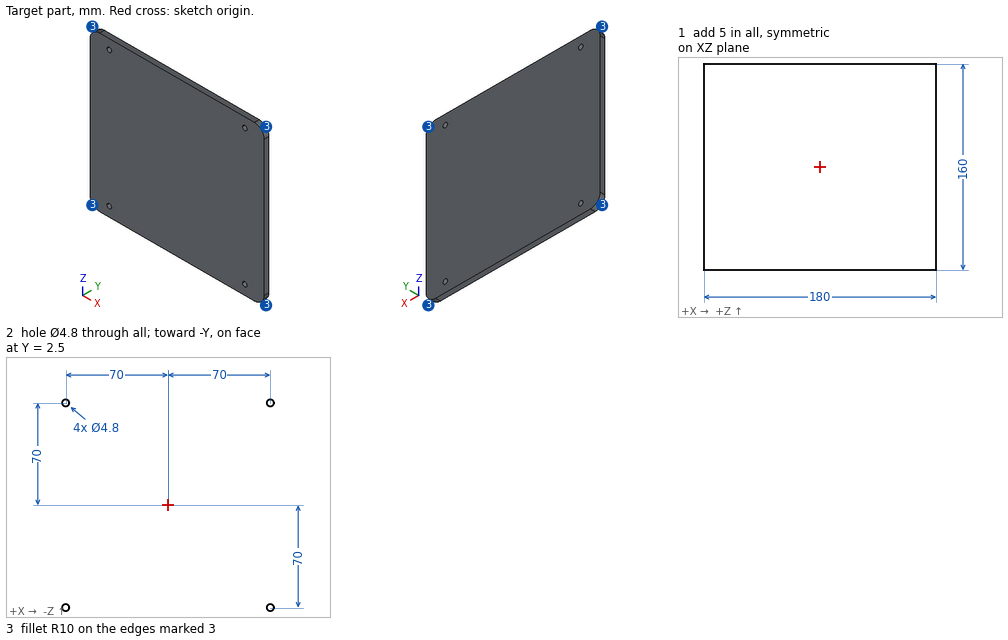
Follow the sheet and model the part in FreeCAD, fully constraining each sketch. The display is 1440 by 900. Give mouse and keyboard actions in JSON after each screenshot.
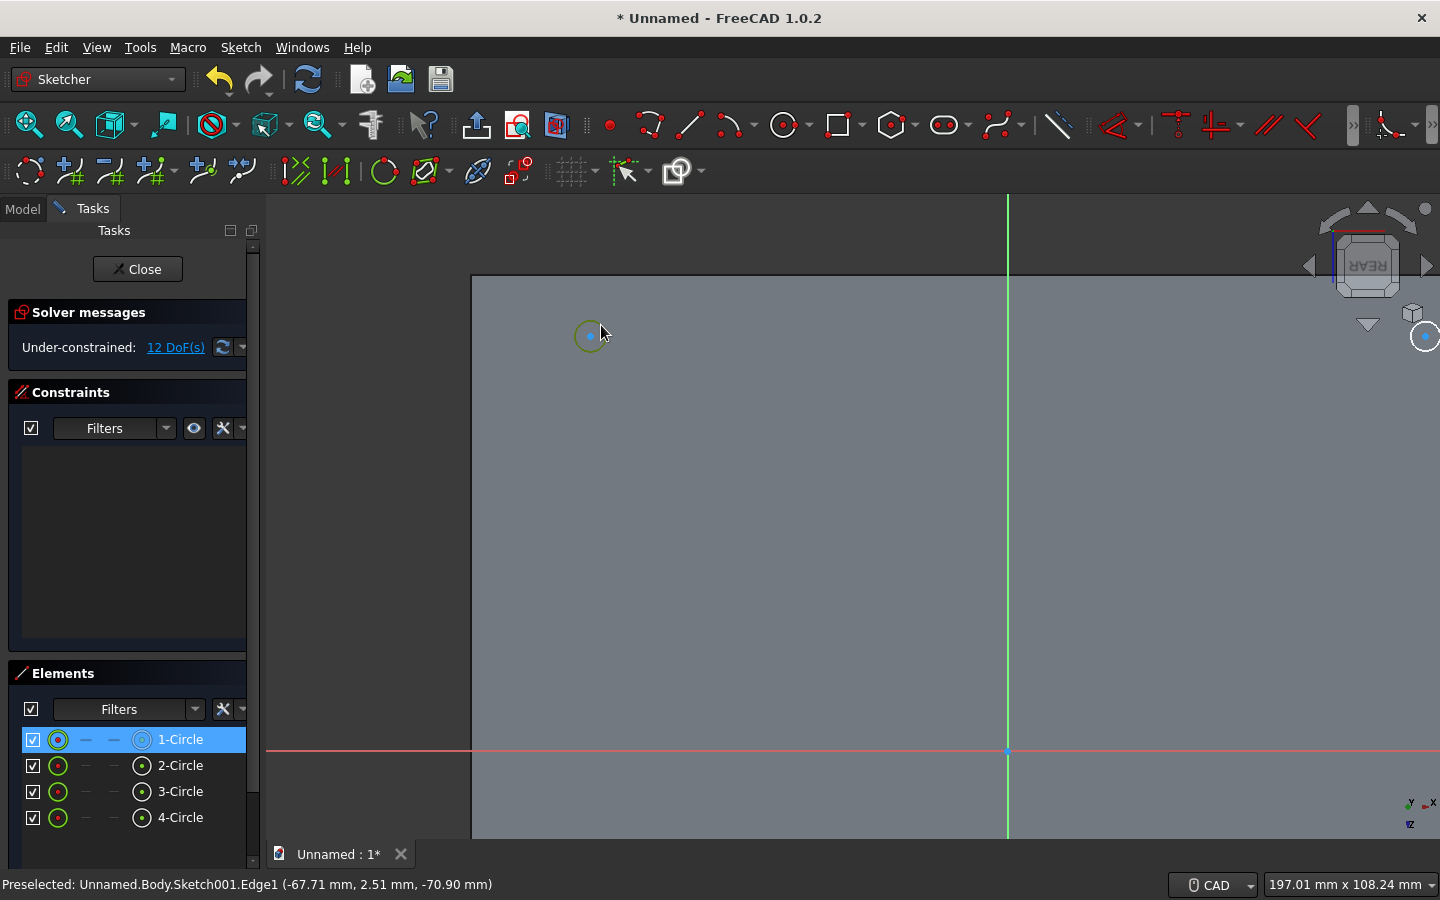
{"action": "scroll", "coordinate": [603, 325], "scroll_direction": "down", "scroll_amount": 4}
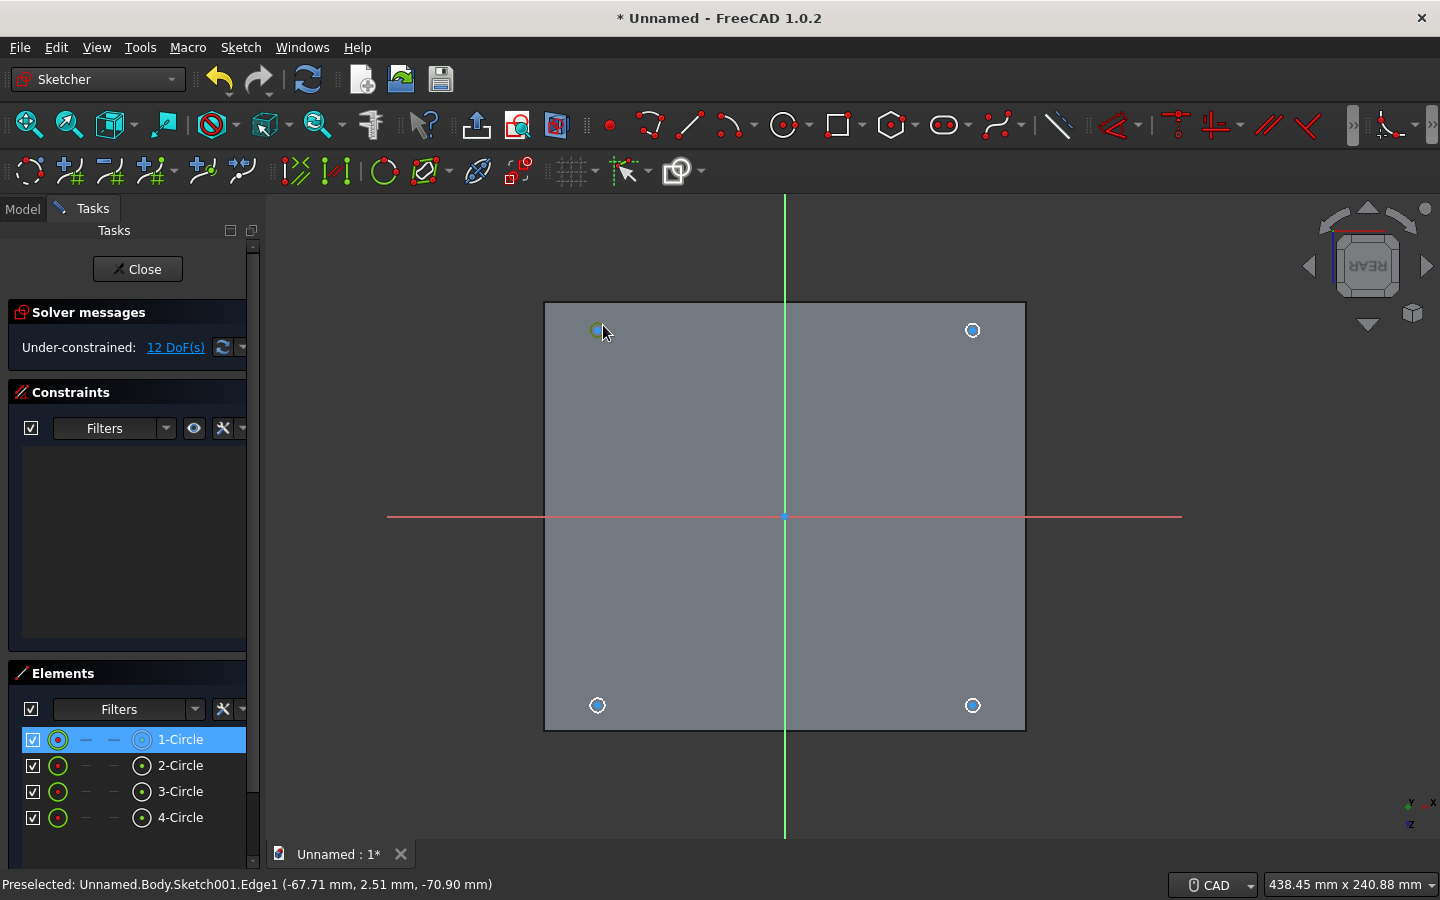
{"action": "scroll", "coordinate": [977, 326], "scroll_direction": "up", "scroll_amount": 4}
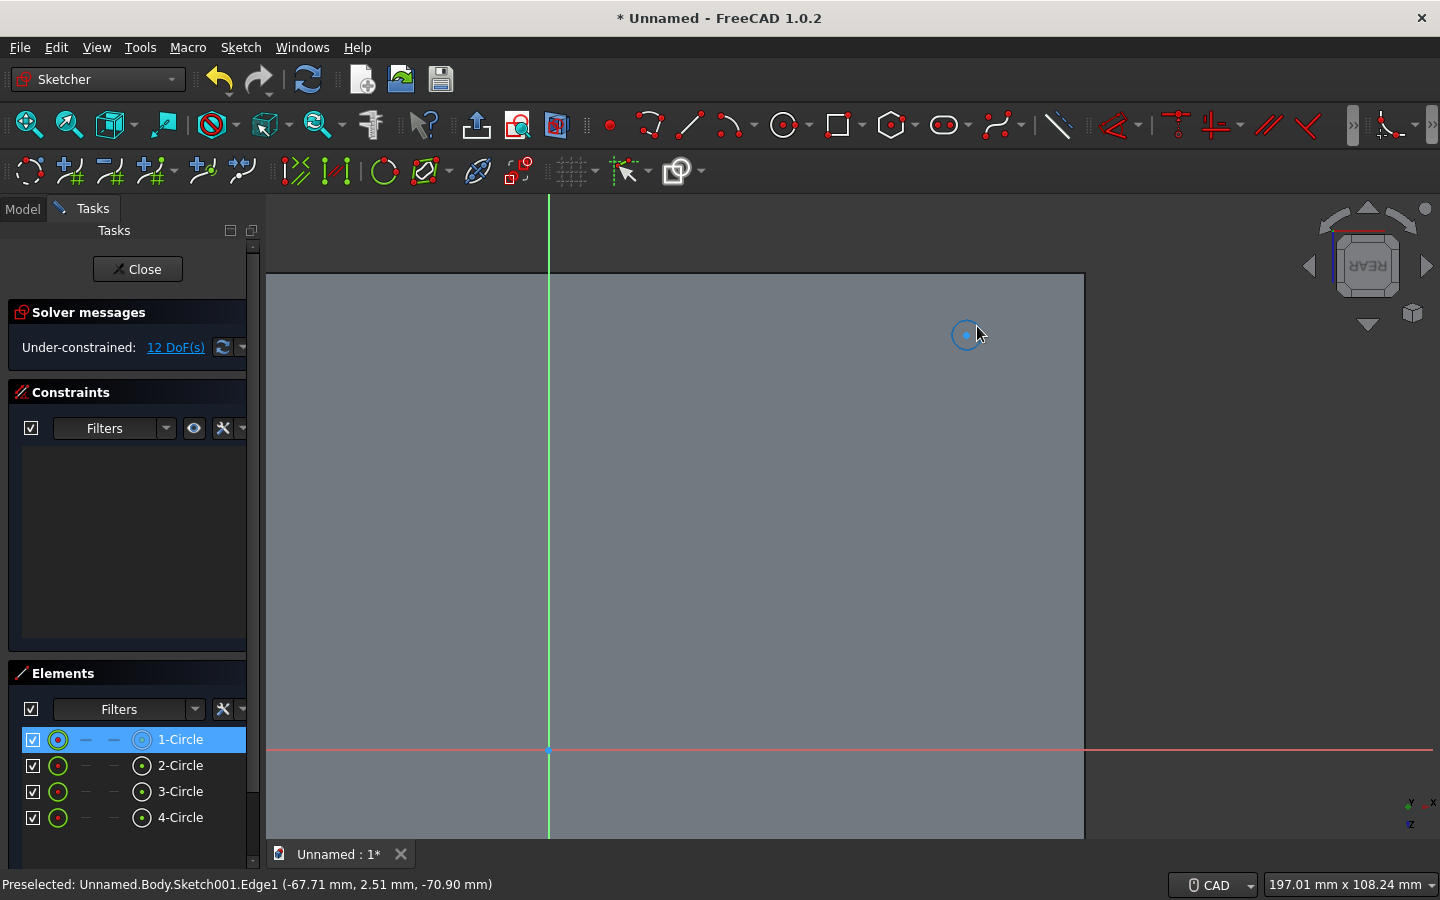
{"action": "left_click", "coordinate": [977, 325]}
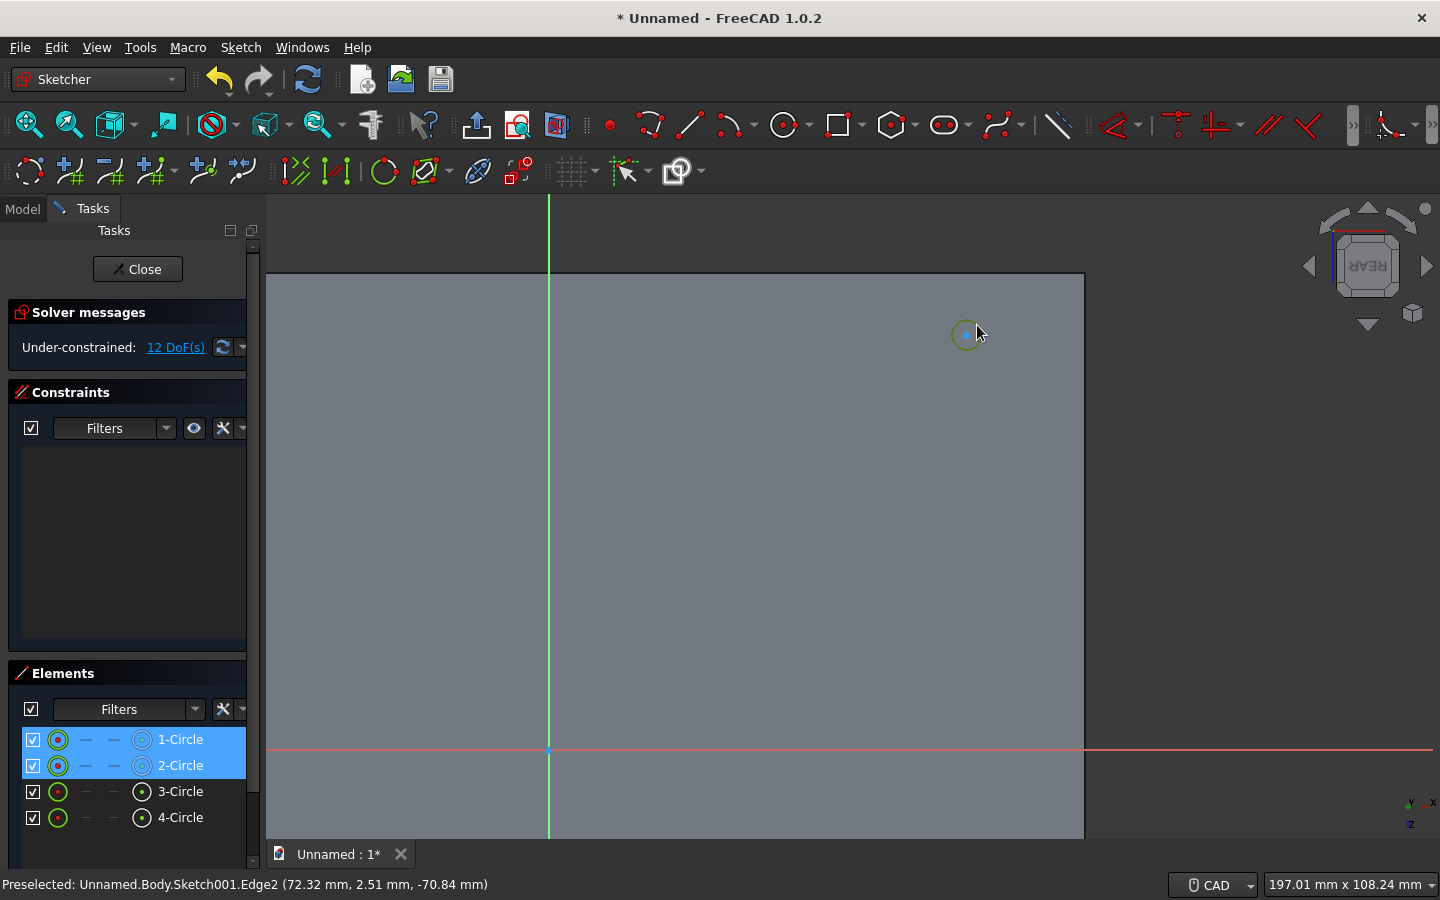
{"action": "scroll", "coordinate": [977, 326], "scroll_direction": "down", "scroll_amount": 4}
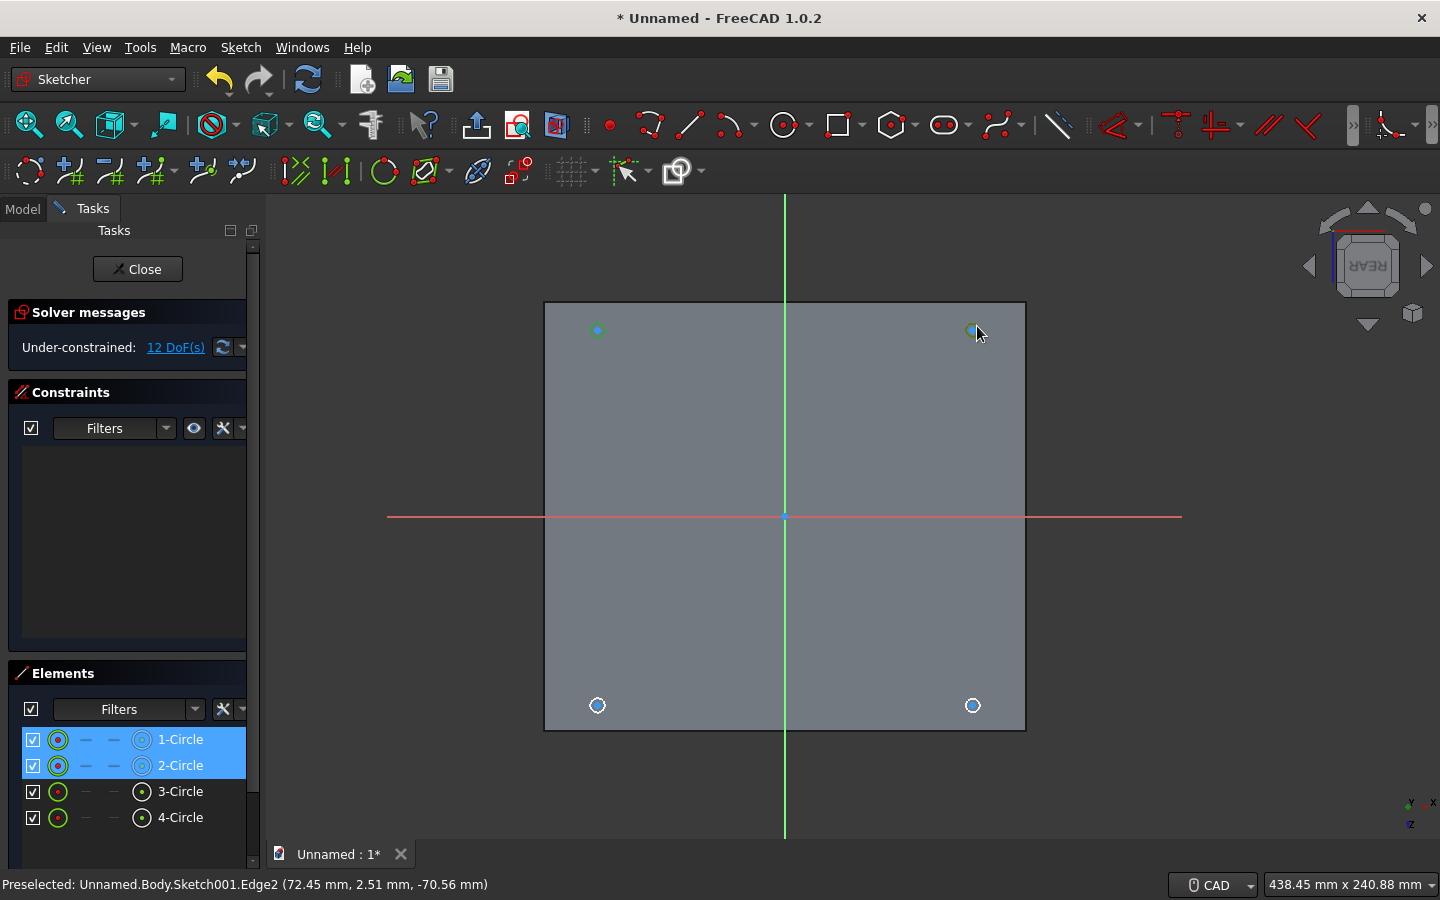
{"action": "scroll", "coordinate": [978, 701], "scroll_direction": "up", "scroll_amount": 4}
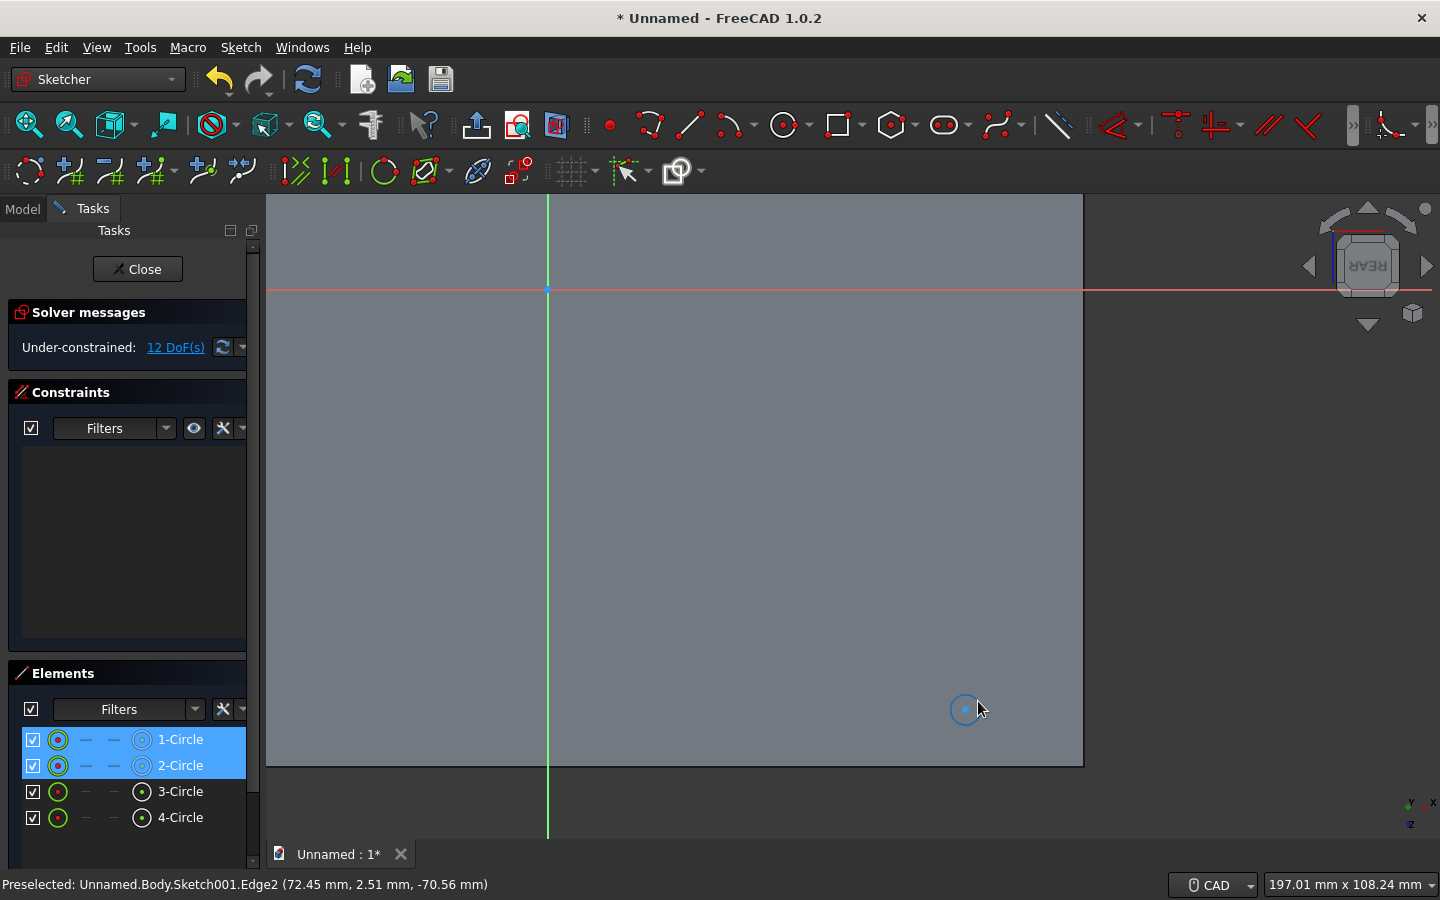
{"action": "left_click", "coordinate": [976, 699]}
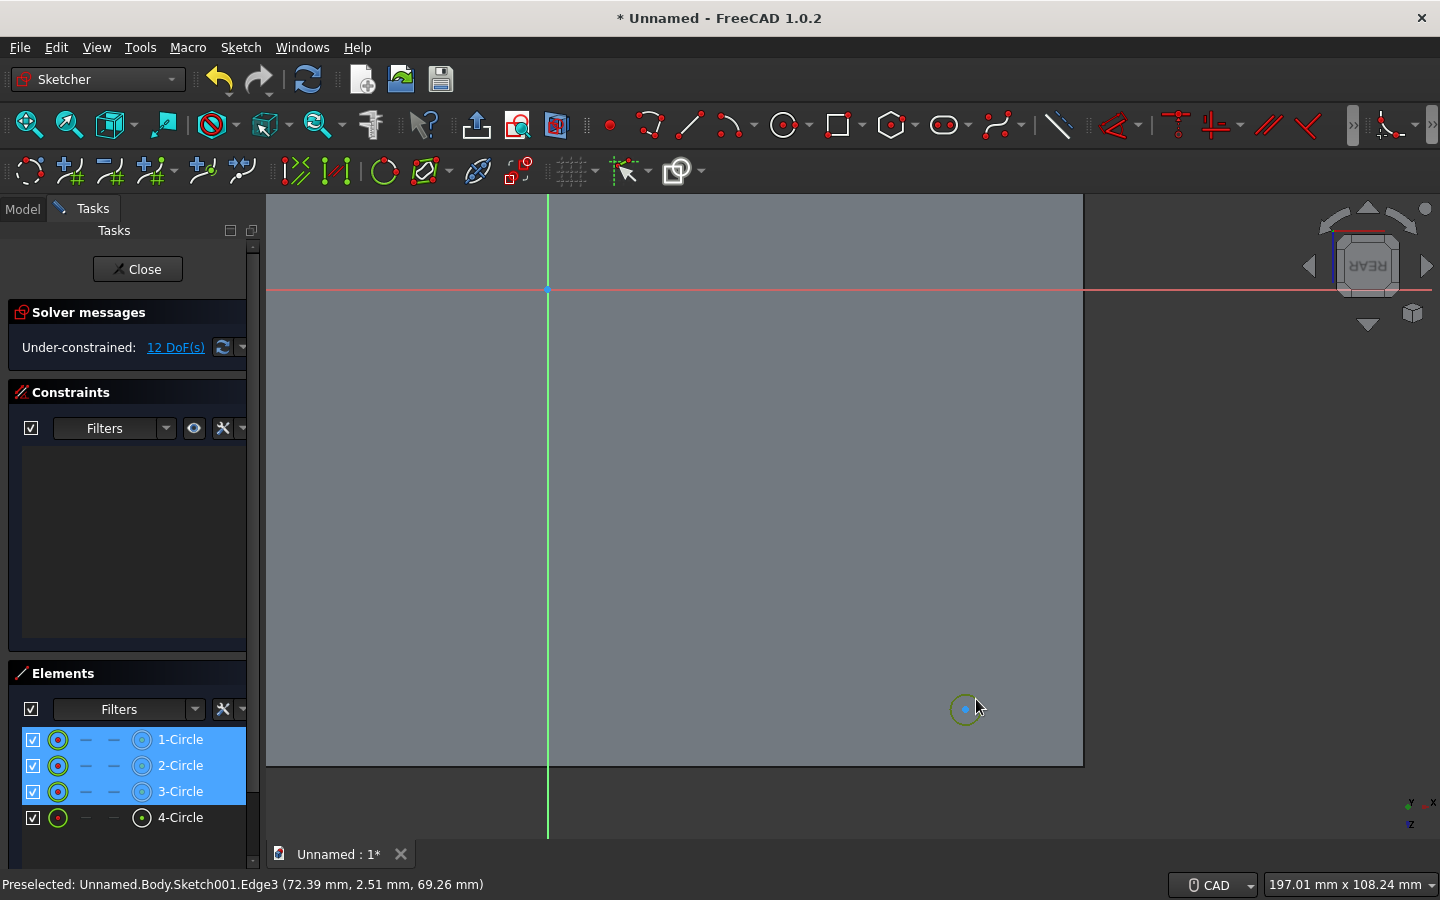
{"action": "scroll", "coordinate": [978, 701], "scroll_direction": "down", "scroll_amount": 4}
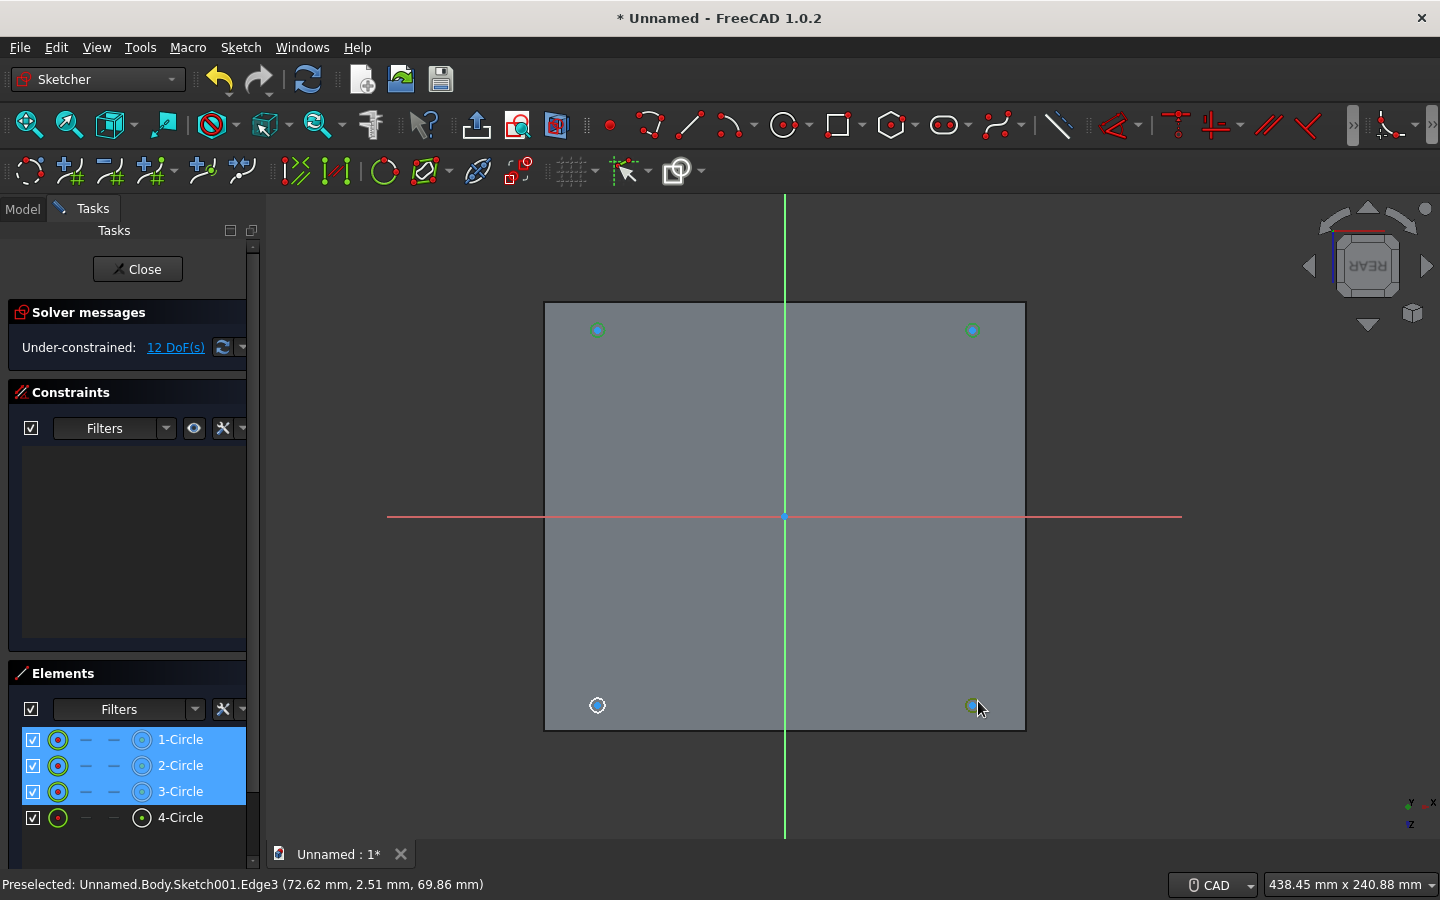
{"action": "scroll", "coordinate": [603, 700], "scroll_direction": "up", "scroll_amount": 4}